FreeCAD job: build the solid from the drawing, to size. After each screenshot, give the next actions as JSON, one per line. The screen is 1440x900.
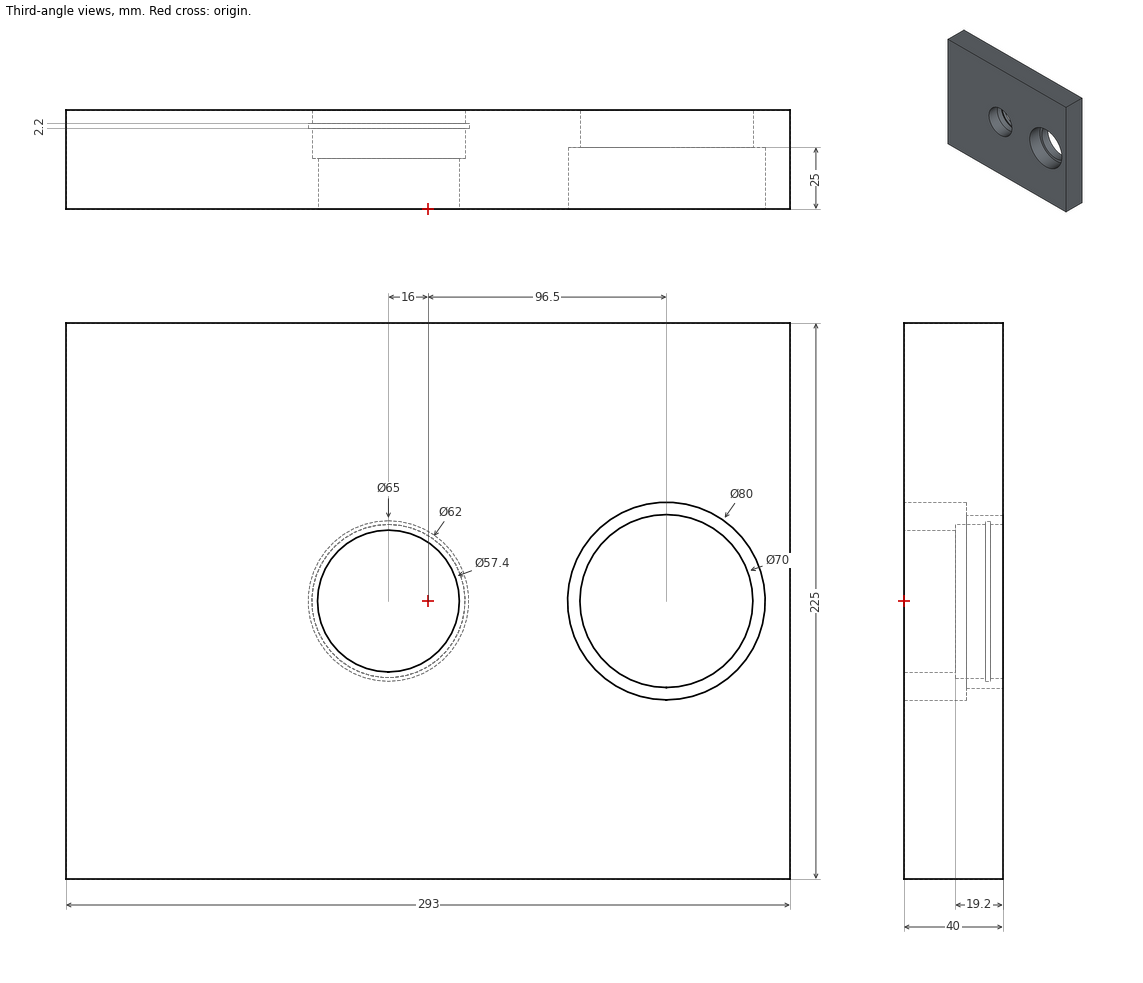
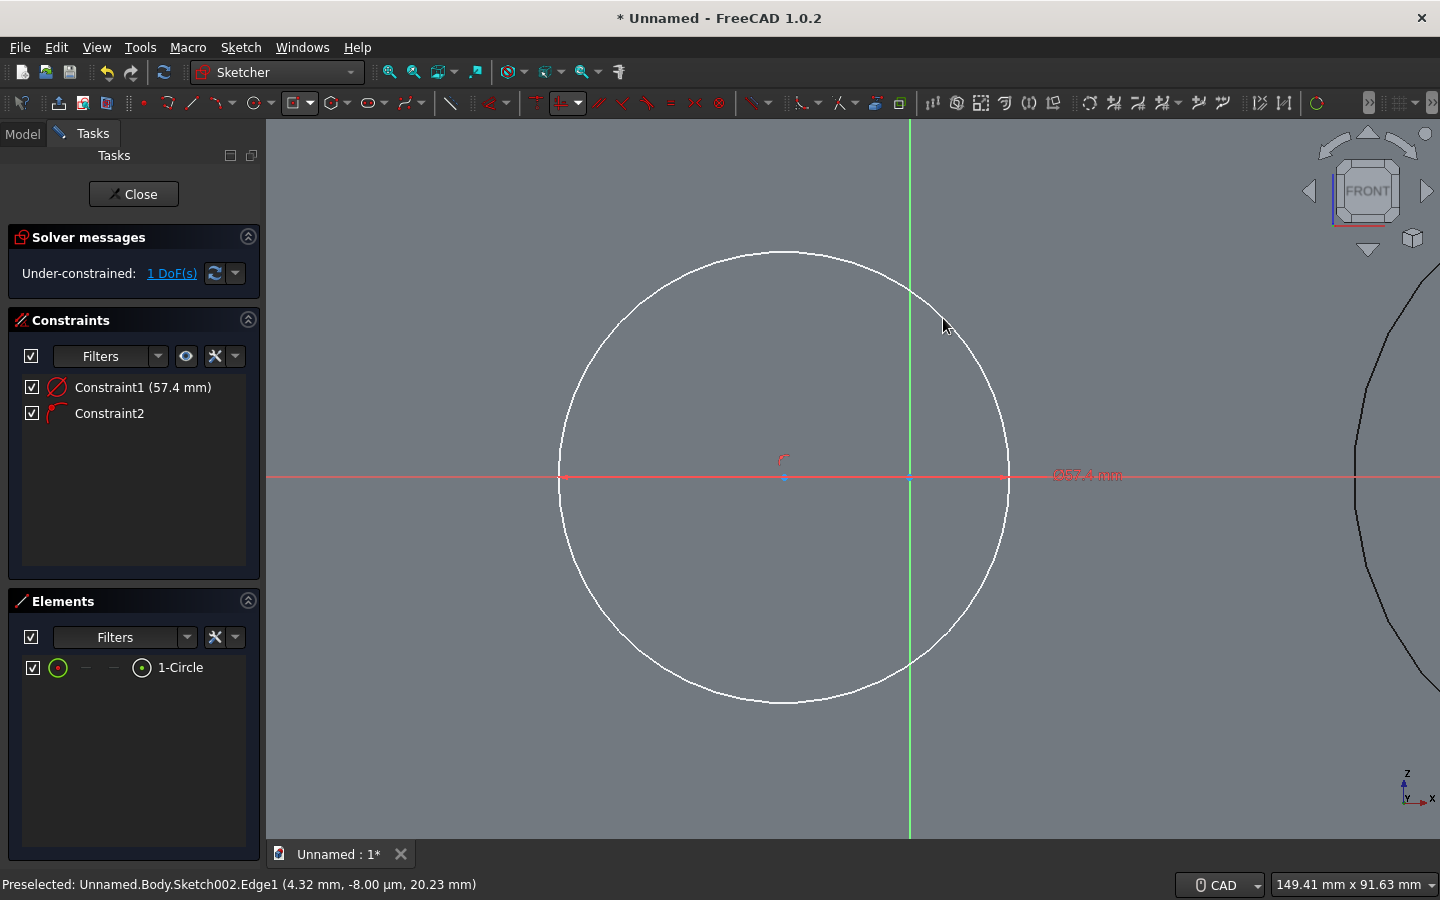
{"action": "left_click", "coordinate": [490, 104]}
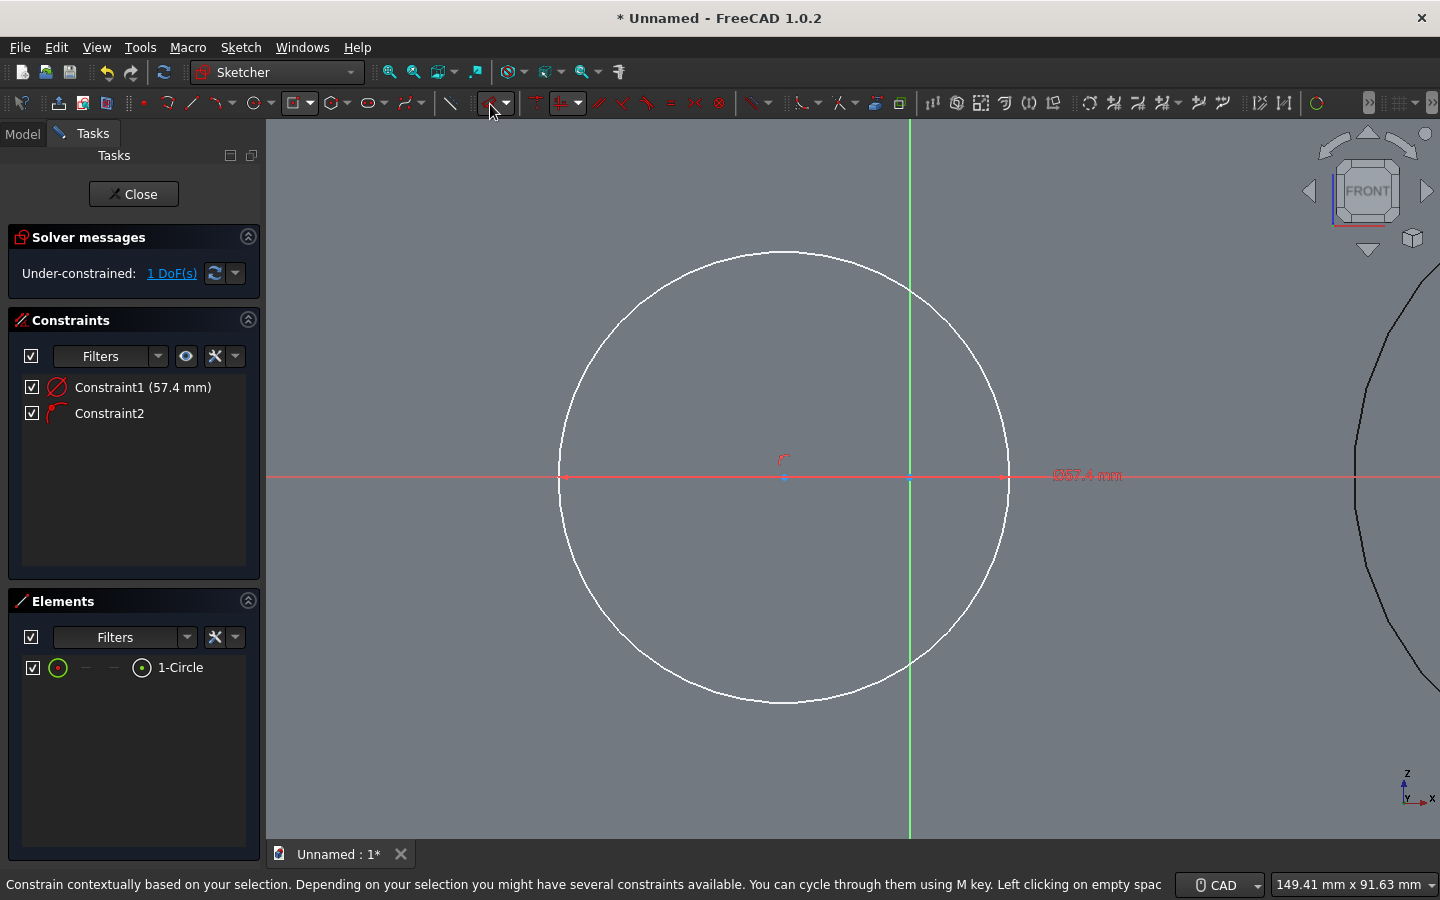
{"action": "left_click", "coordinate": [784, 477]}
{"action": "left_click", "coordinate": [847, 511]}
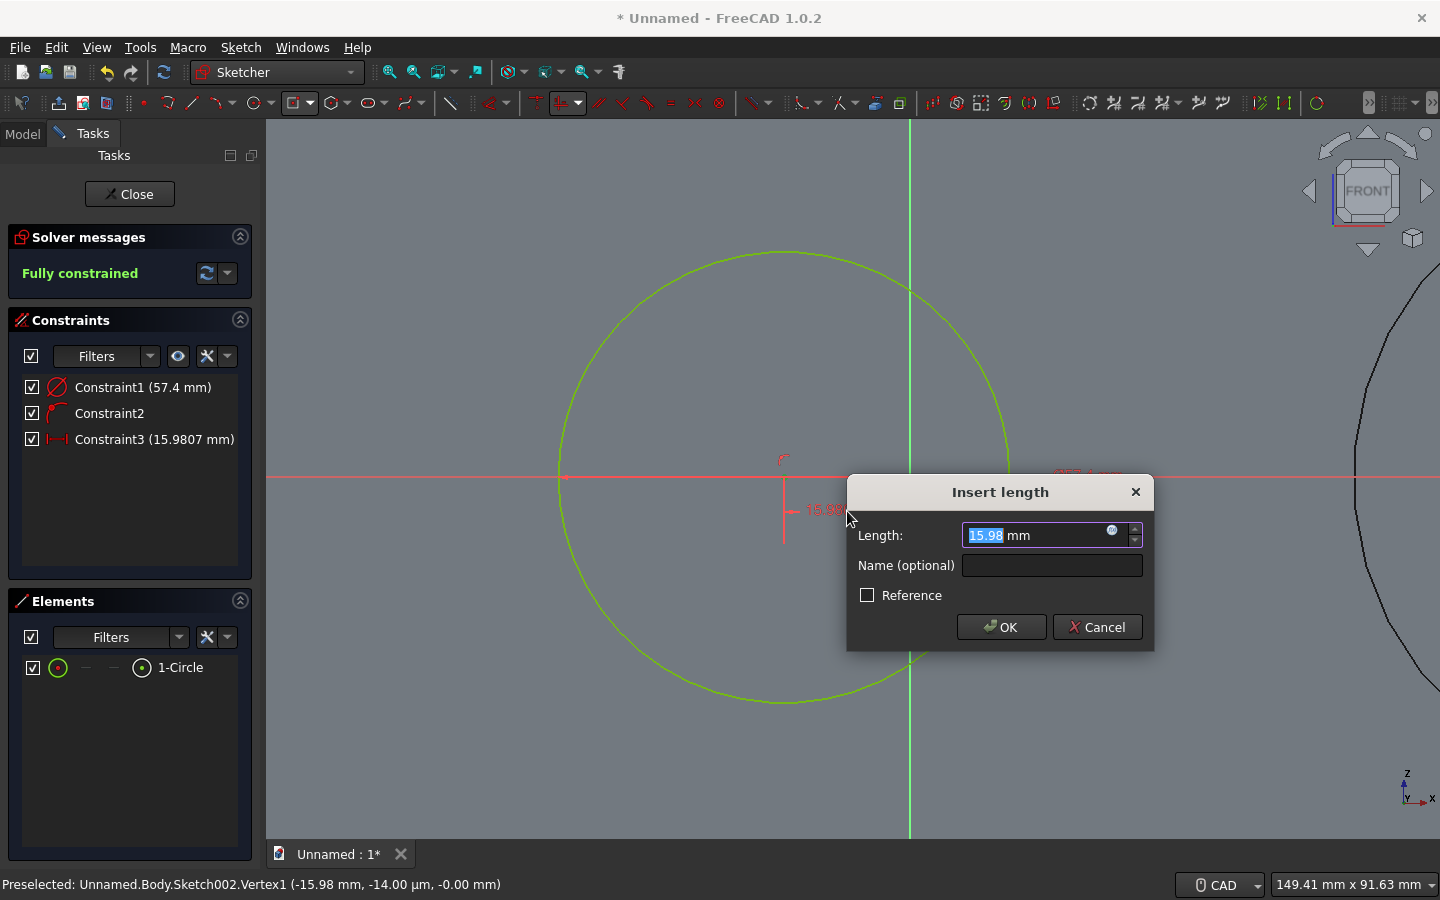
{"action": "type", "text": "16"}
{"action": "key", "text": "Return"}
{"action": "key", "text": "Escape"}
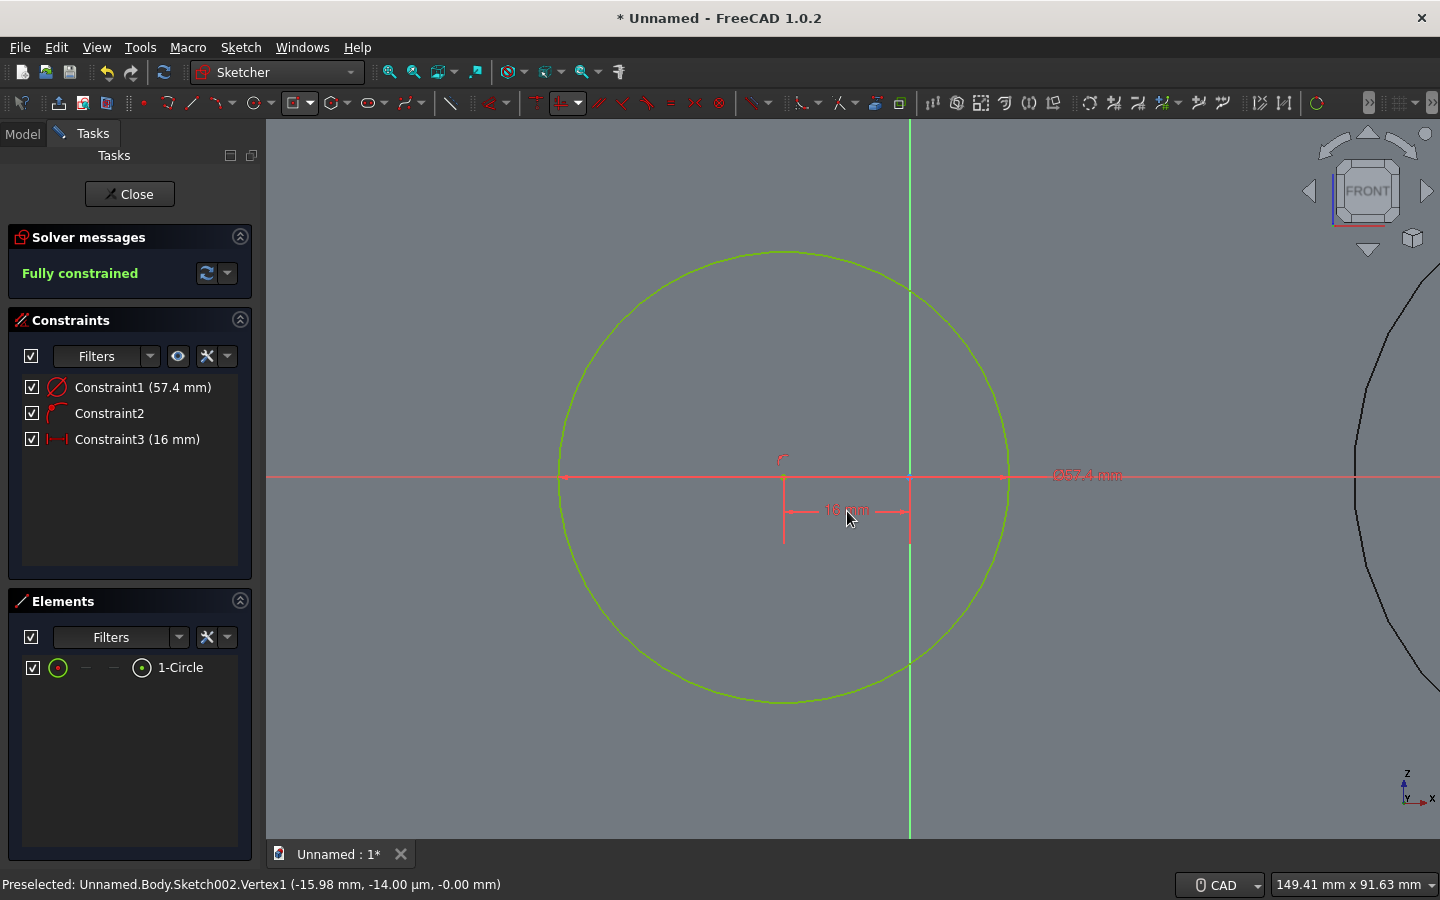
{"action": "left_click", "coordinate": [130, 194]}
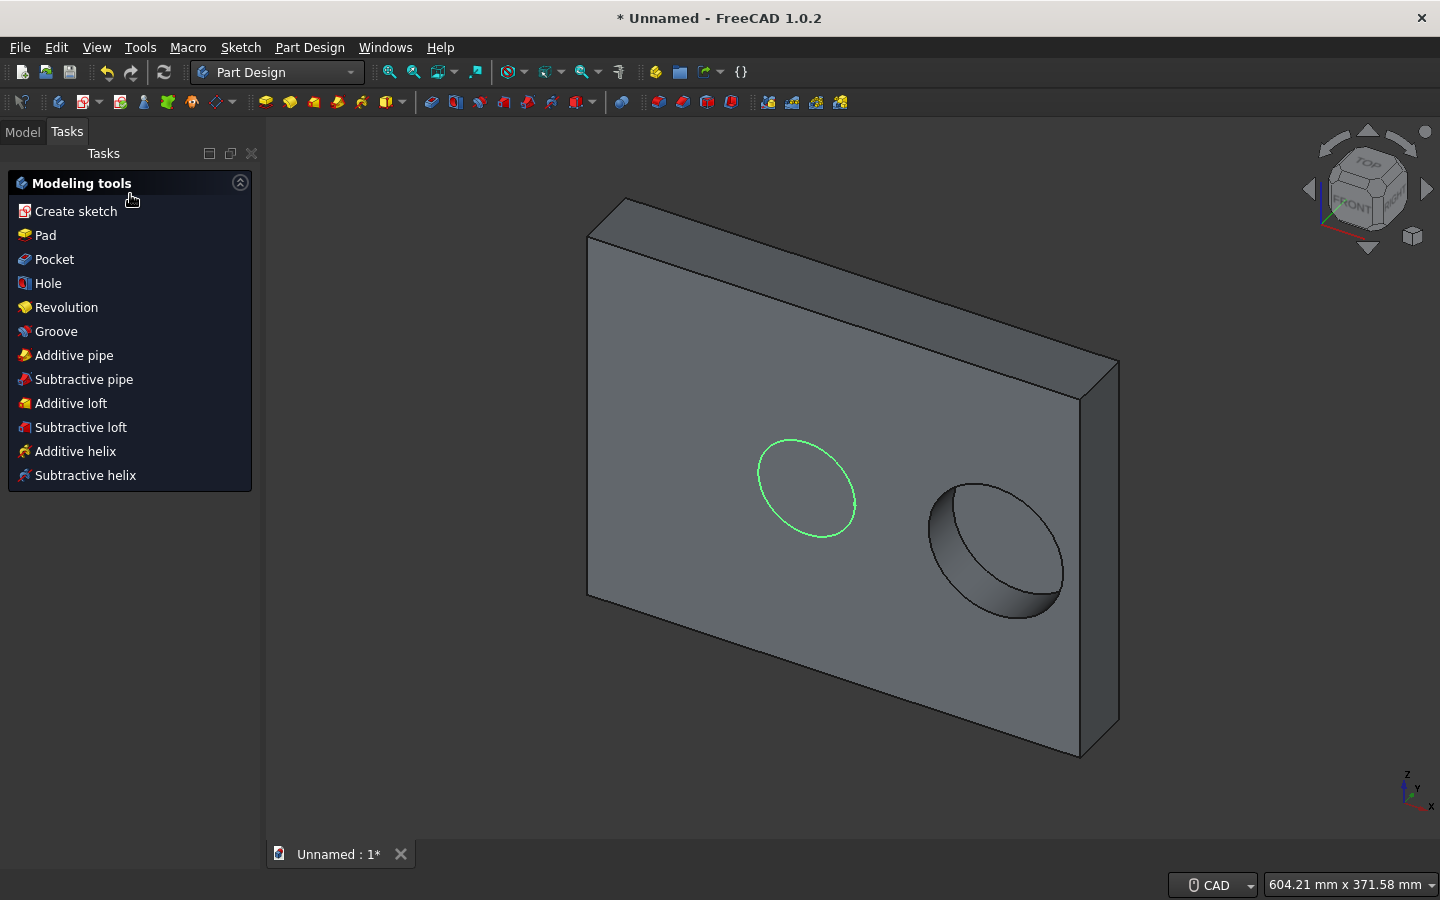
{"action": "left_click", "coordinate": [432, 102]}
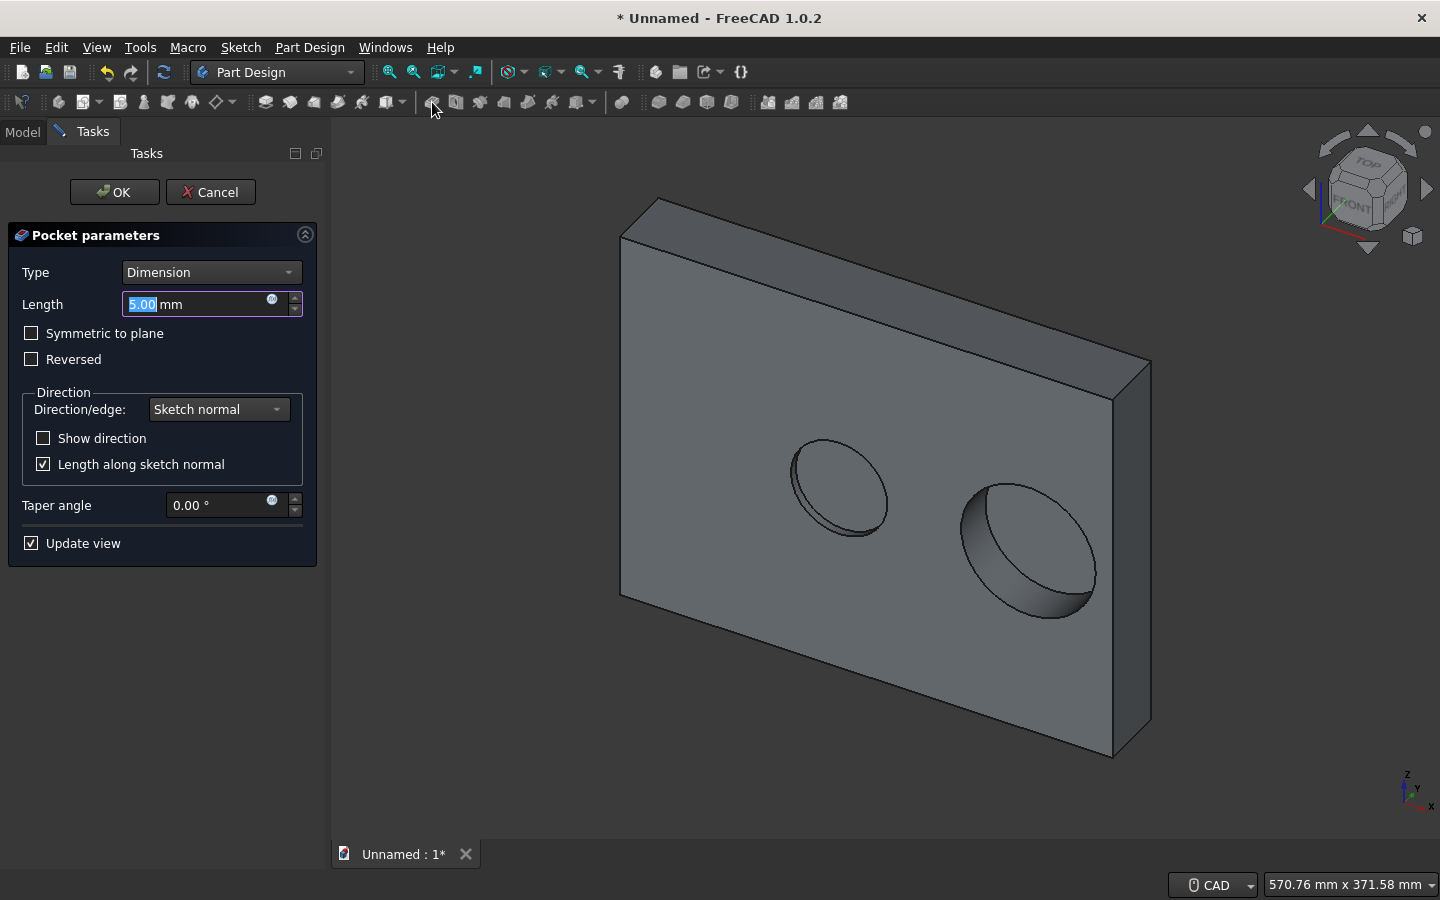
{"action": "left_click", "coordinate": [212, 272]}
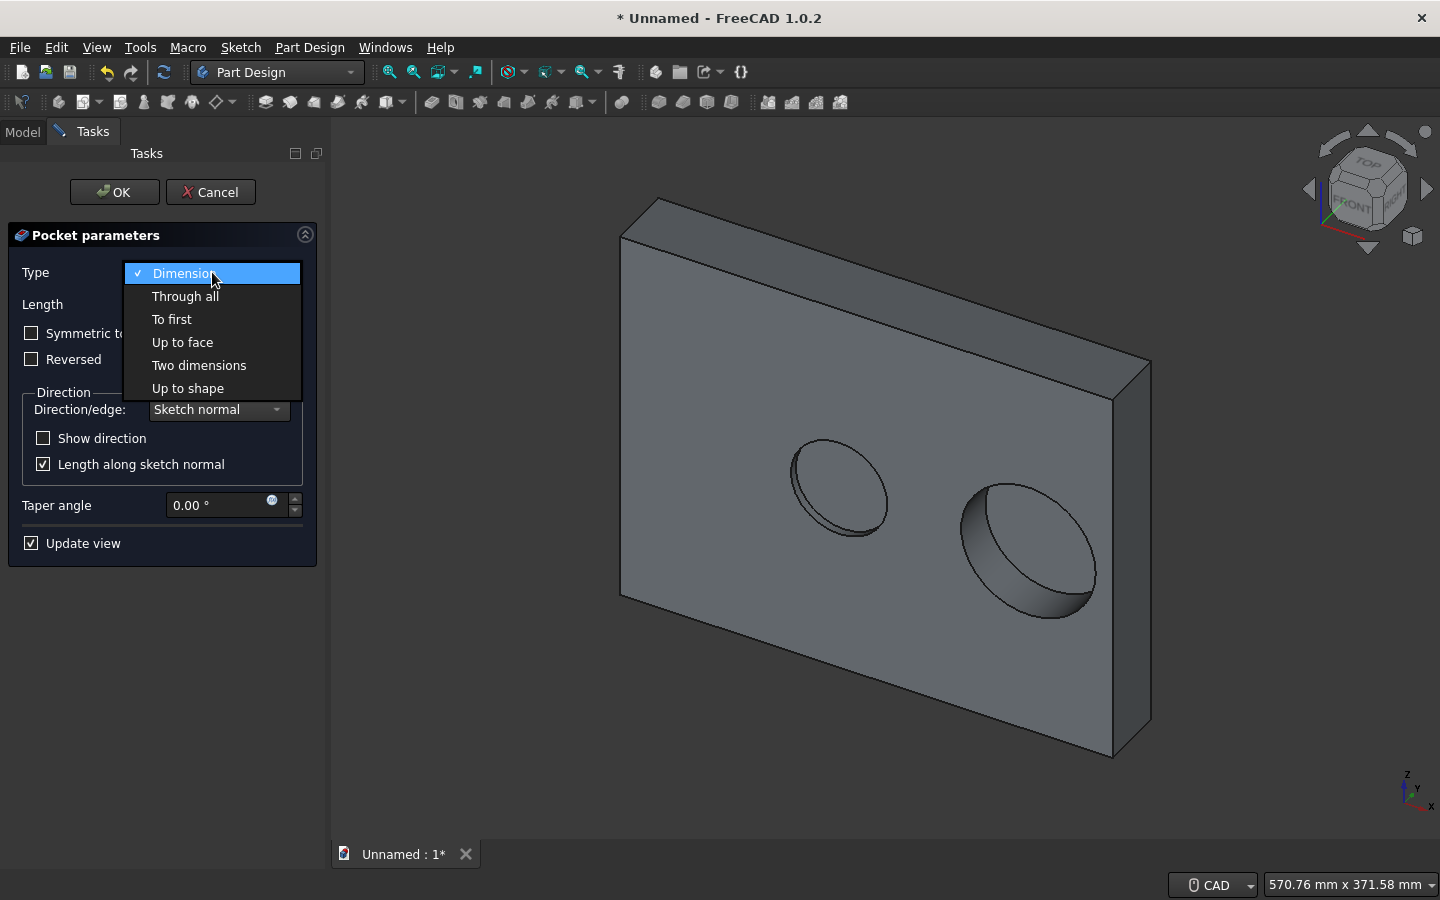
{"action": "left_click", "coordinate": [212, 296]}